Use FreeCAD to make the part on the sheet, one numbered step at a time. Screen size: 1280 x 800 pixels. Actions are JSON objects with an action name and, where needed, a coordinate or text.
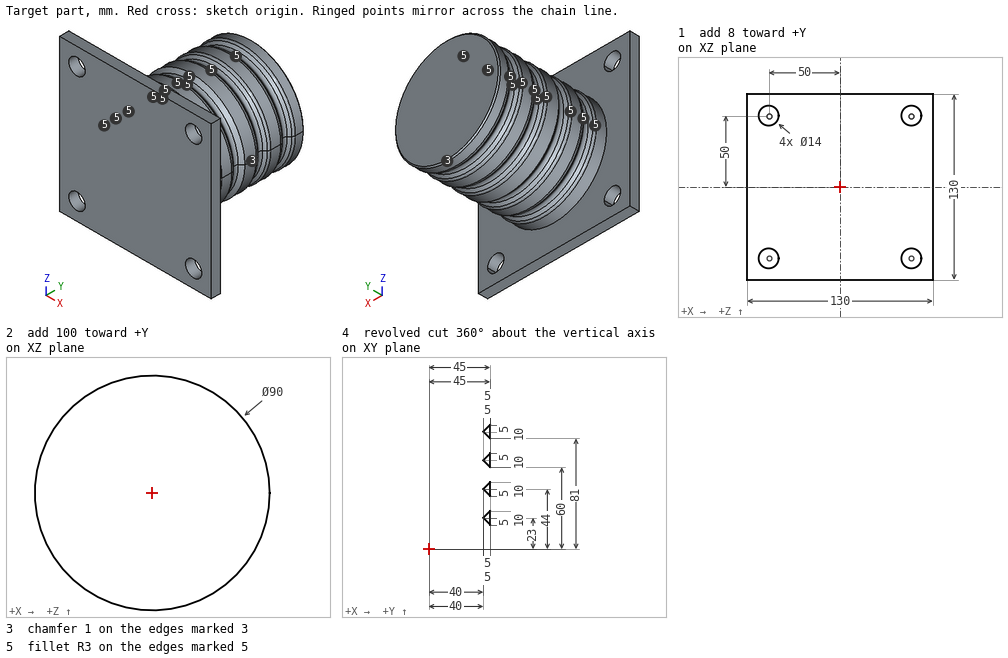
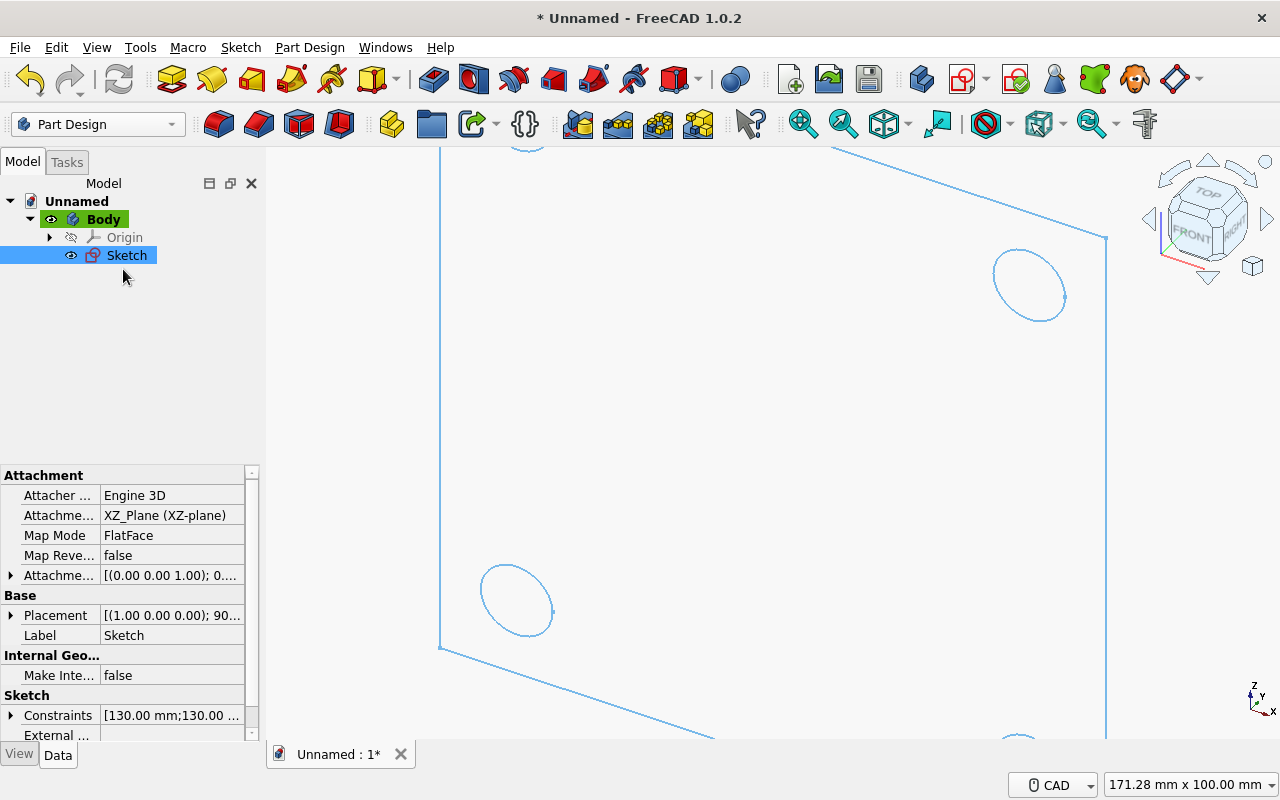
{"action": "left_click", "coordinate": [172, 80]}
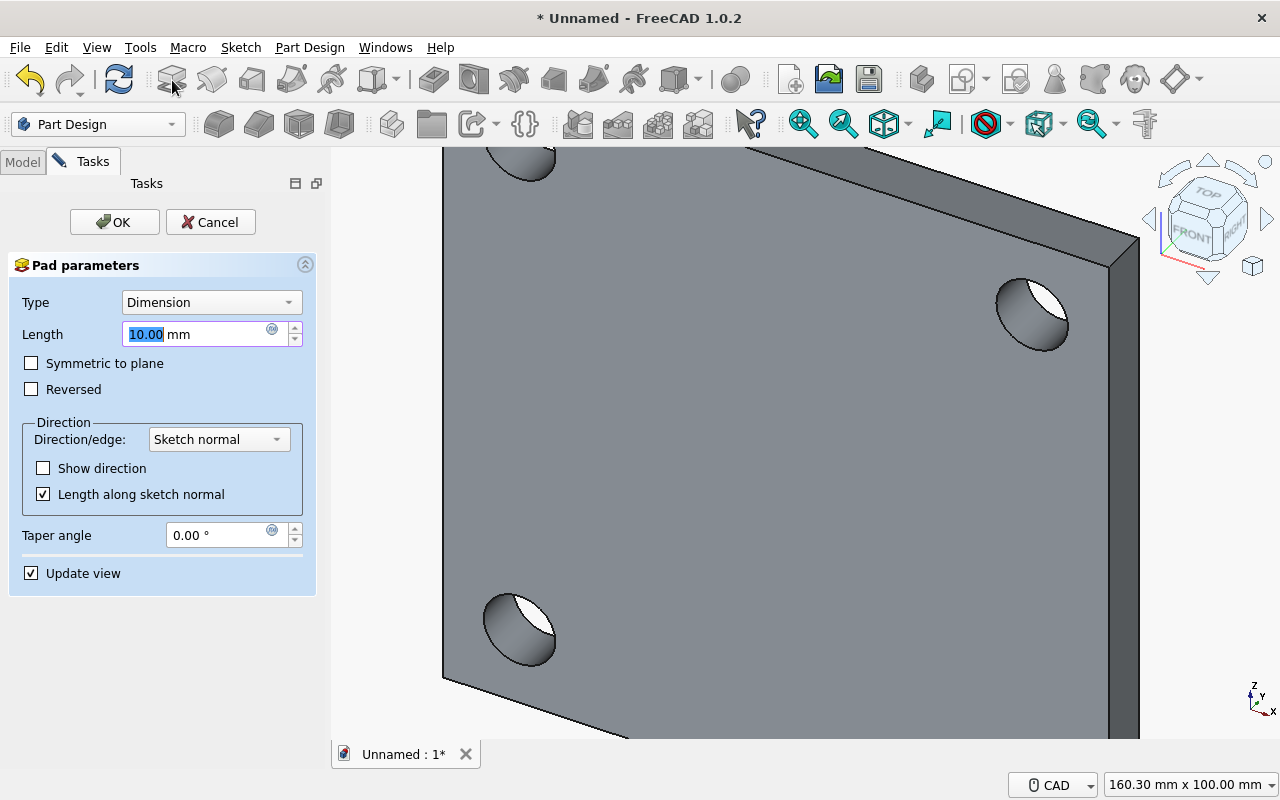
{"action": "type", "text": "8"}
{"action": "key", "text": "Tab"}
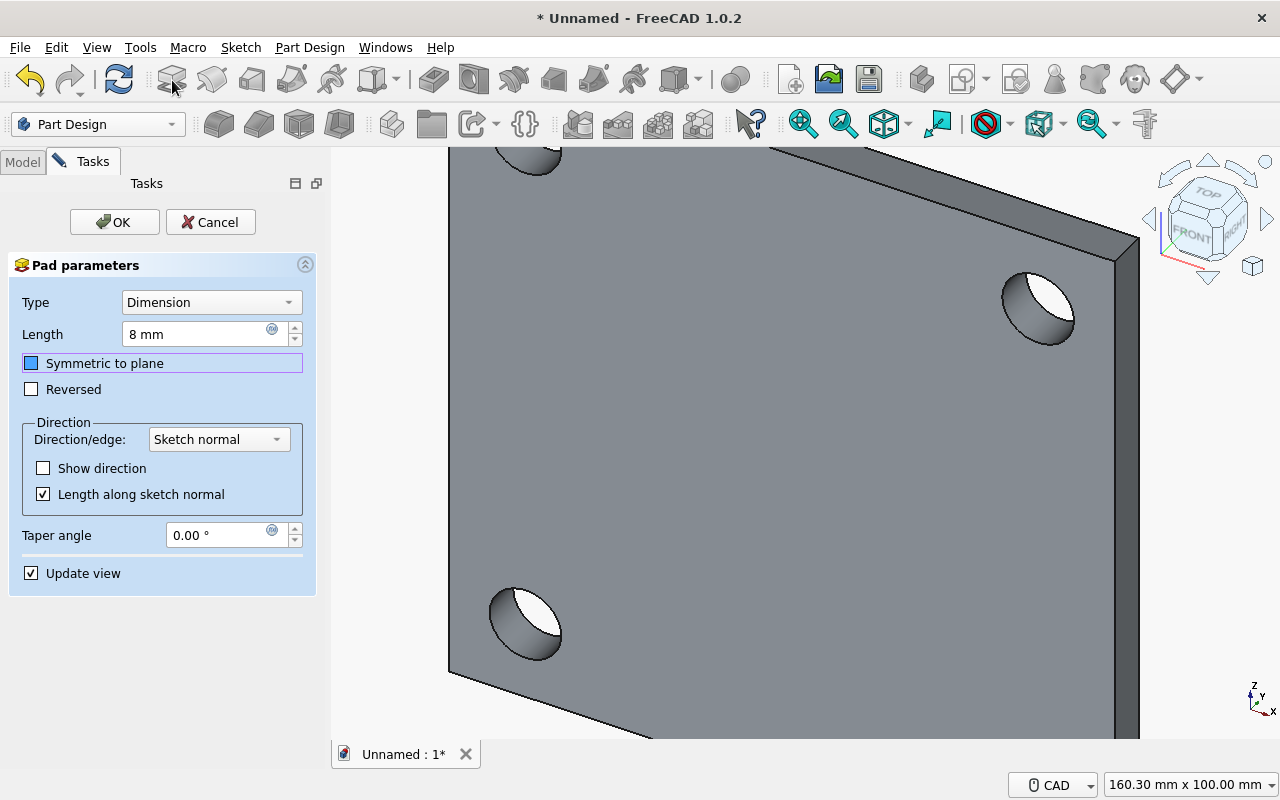
{"action": "left_click", "coordinate": [30, 389]}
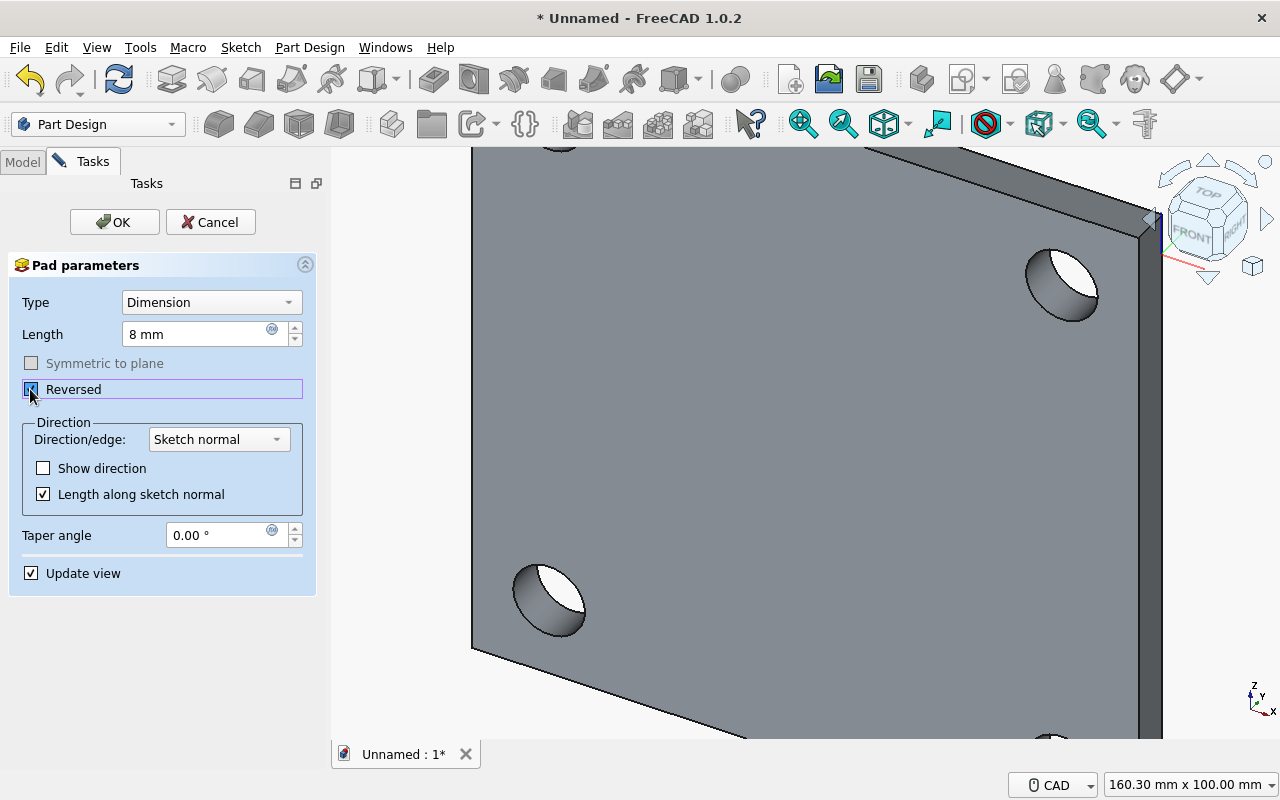
{"action": "left_click", "coordinate": [115, 222]}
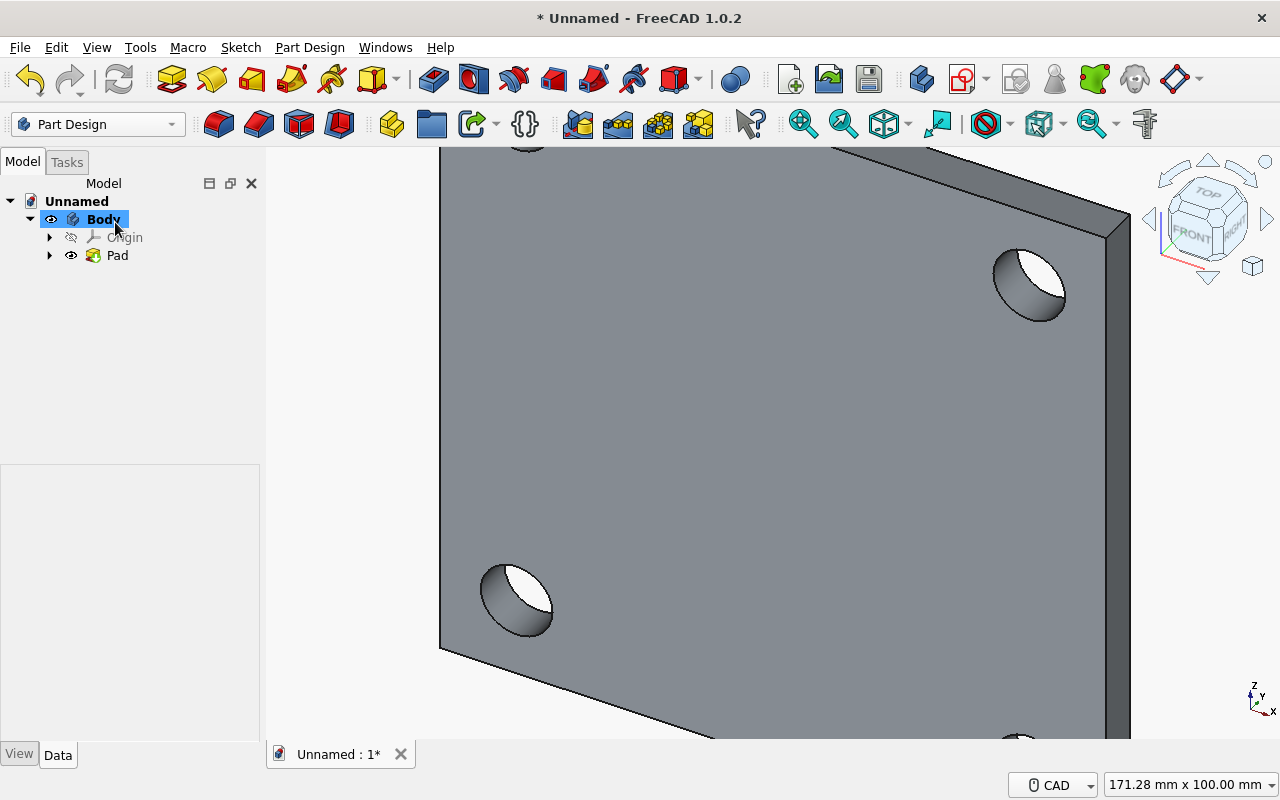
{"action": "left_click", "coordinate": [804, 124]}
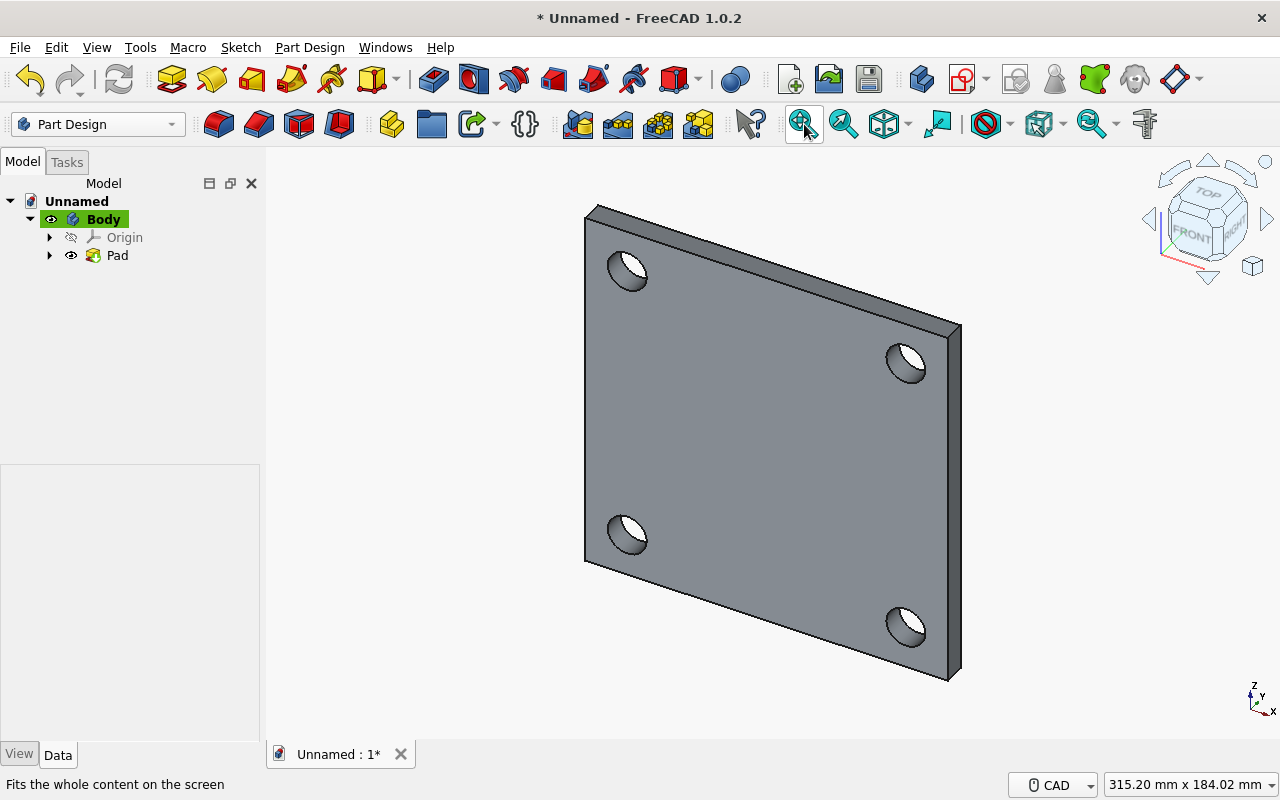
{"action": "left_click", "coordinate": [962, 80]}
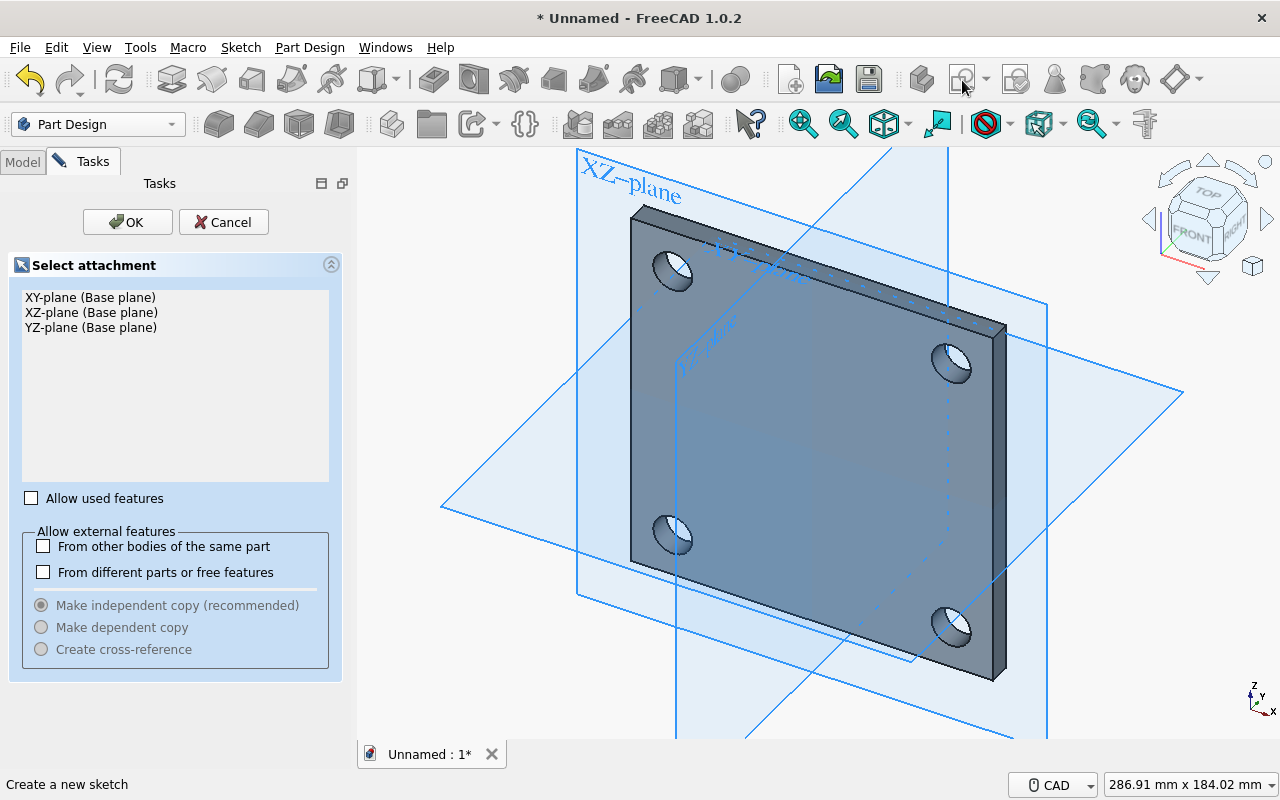
{"action": "left_click", "coordinate": [82, 312]}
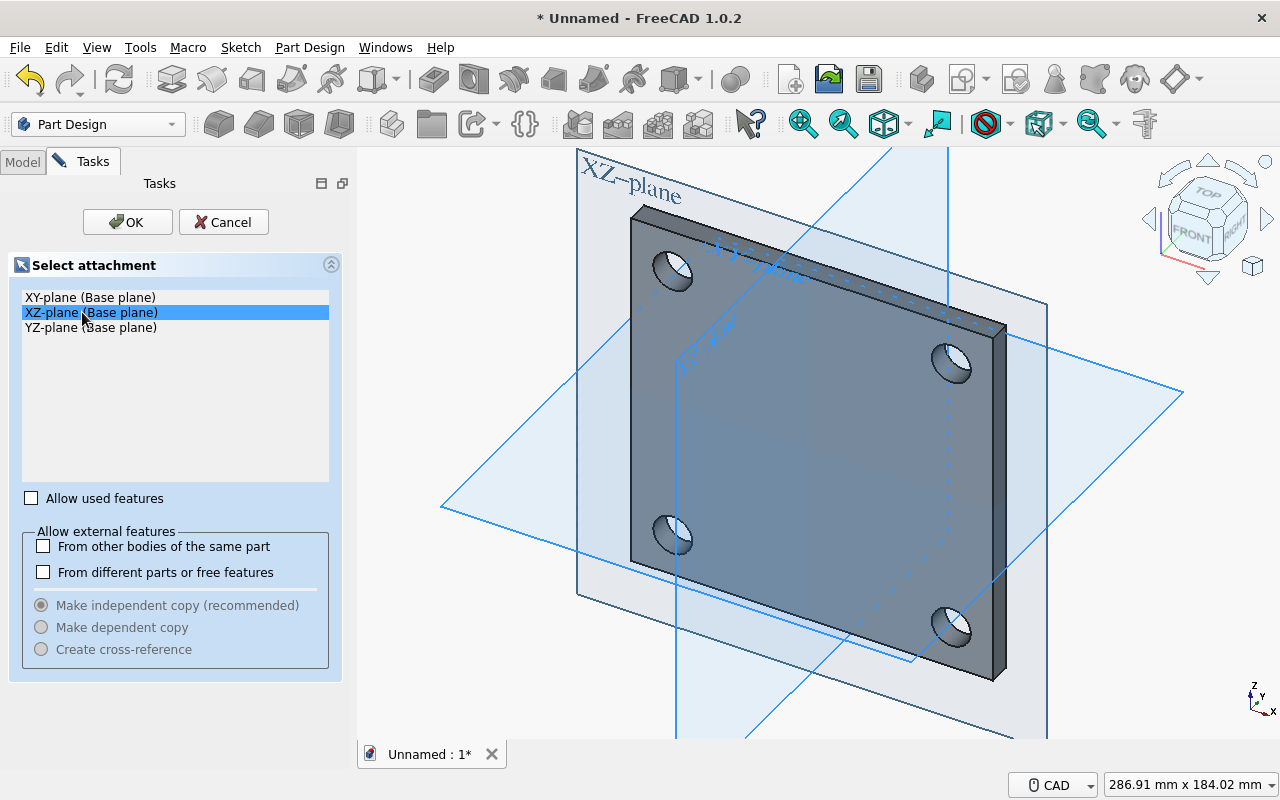
{"action": "left_click", "coordinate": [128, 222]}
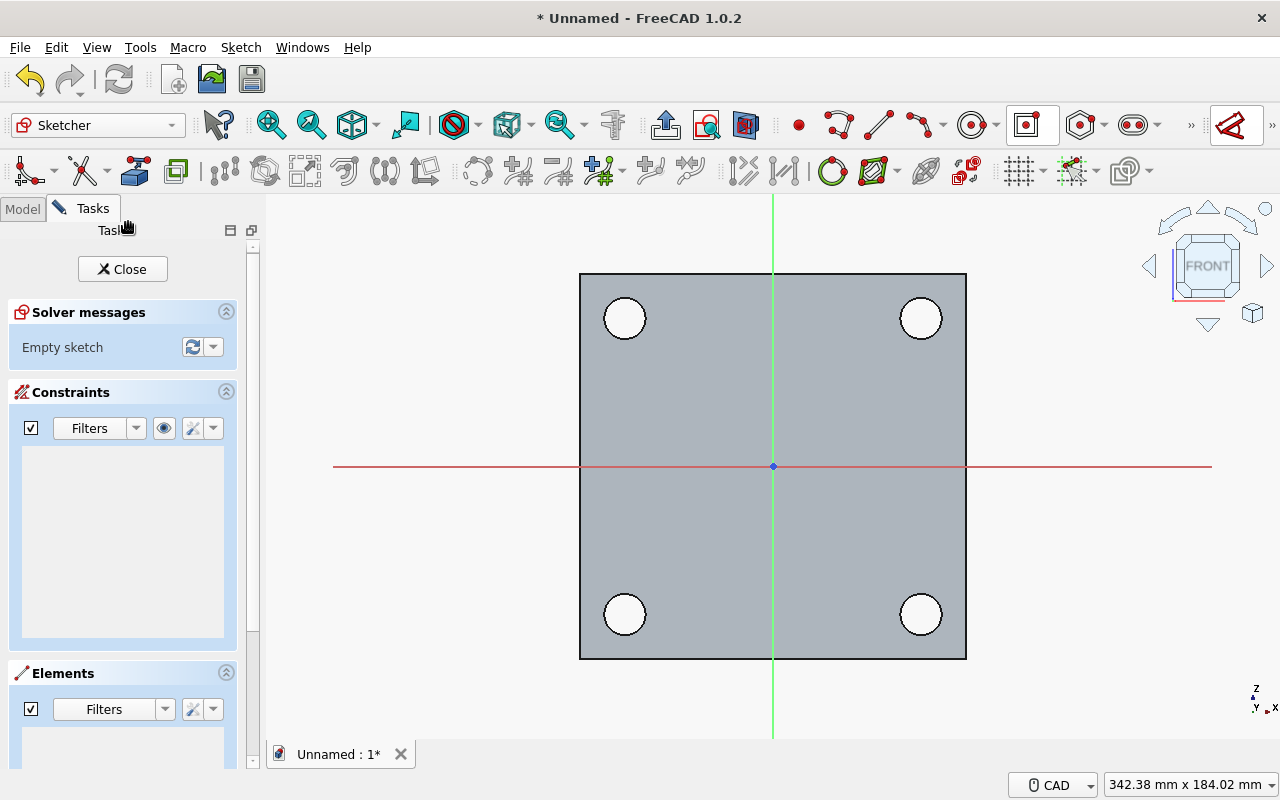
{"action": "left_click", "coordinate": [972, 126]}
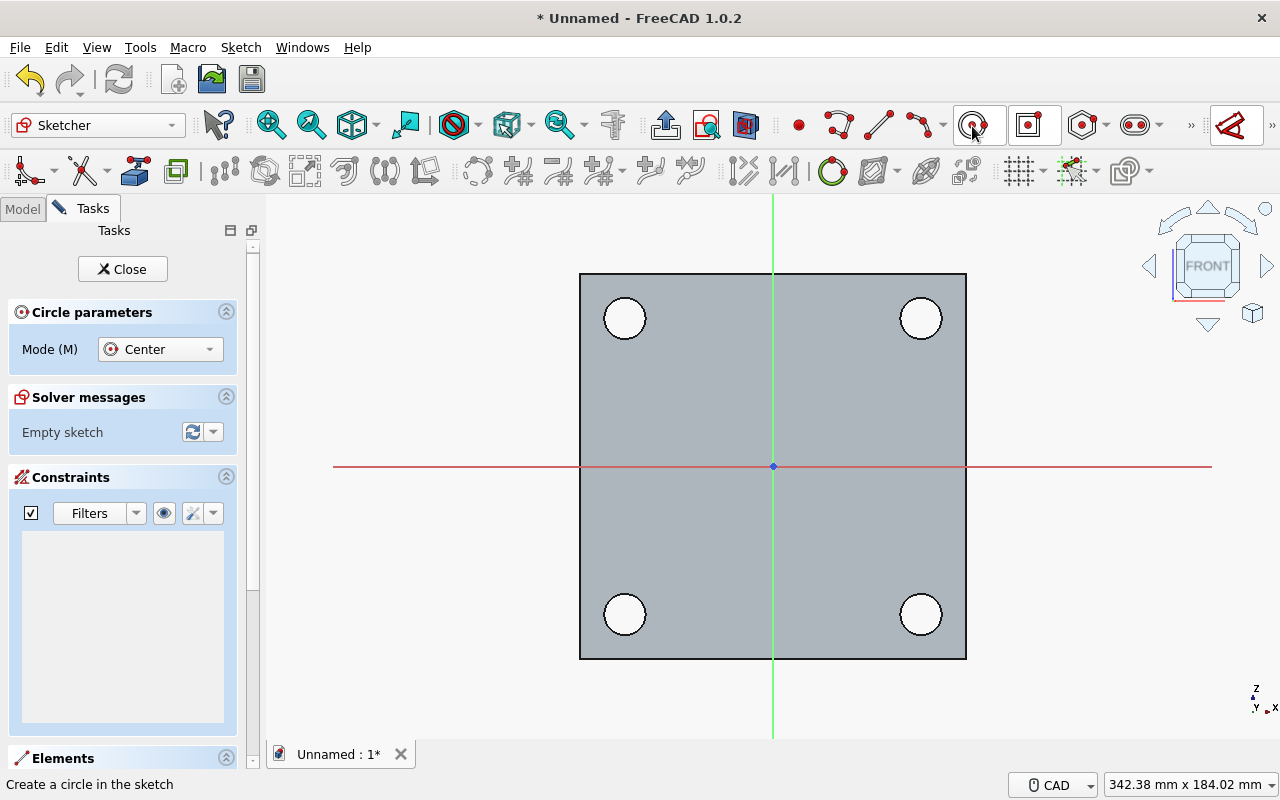
{"action": "left_click", "coordinate": [773, 467]}
{"action": "mouse_move", "coordinate": [867, 372]}